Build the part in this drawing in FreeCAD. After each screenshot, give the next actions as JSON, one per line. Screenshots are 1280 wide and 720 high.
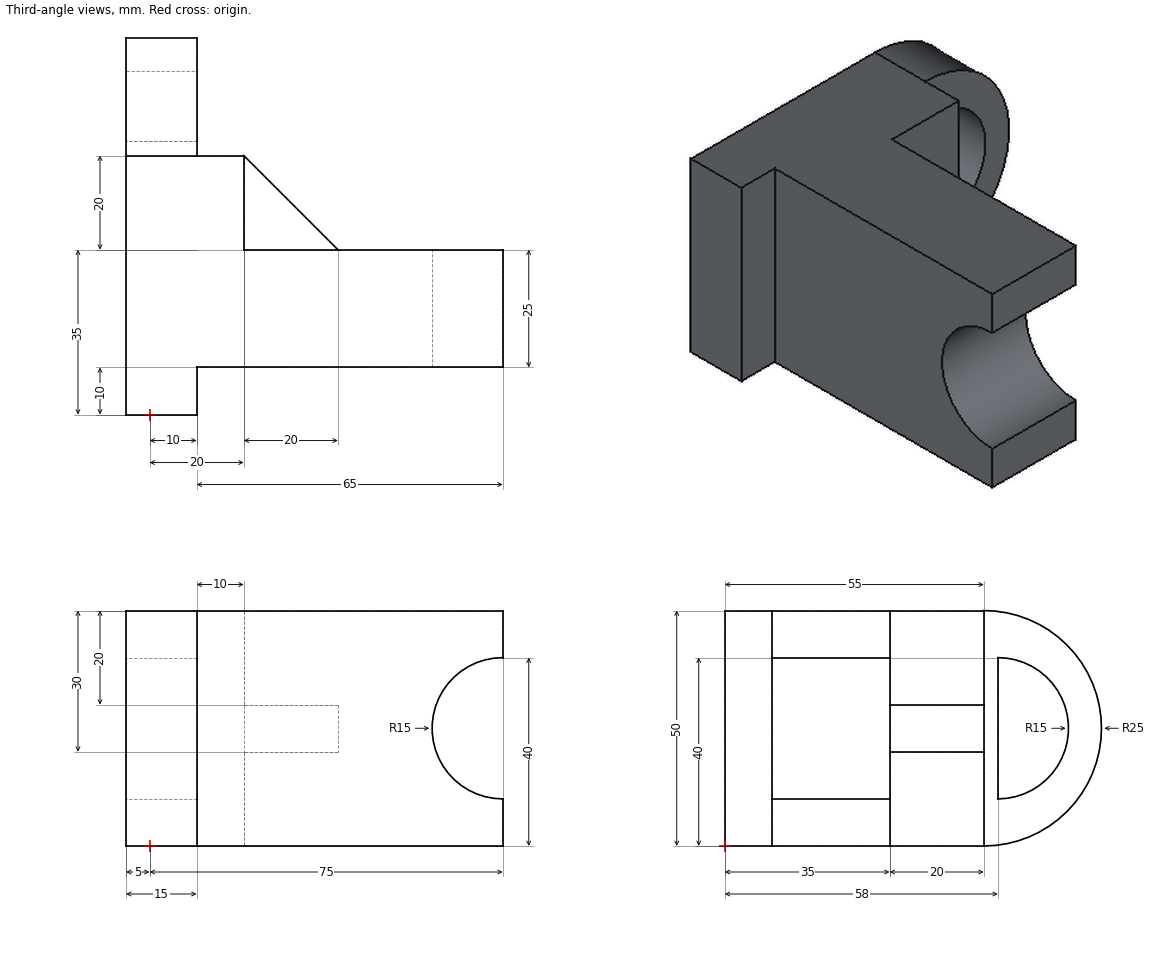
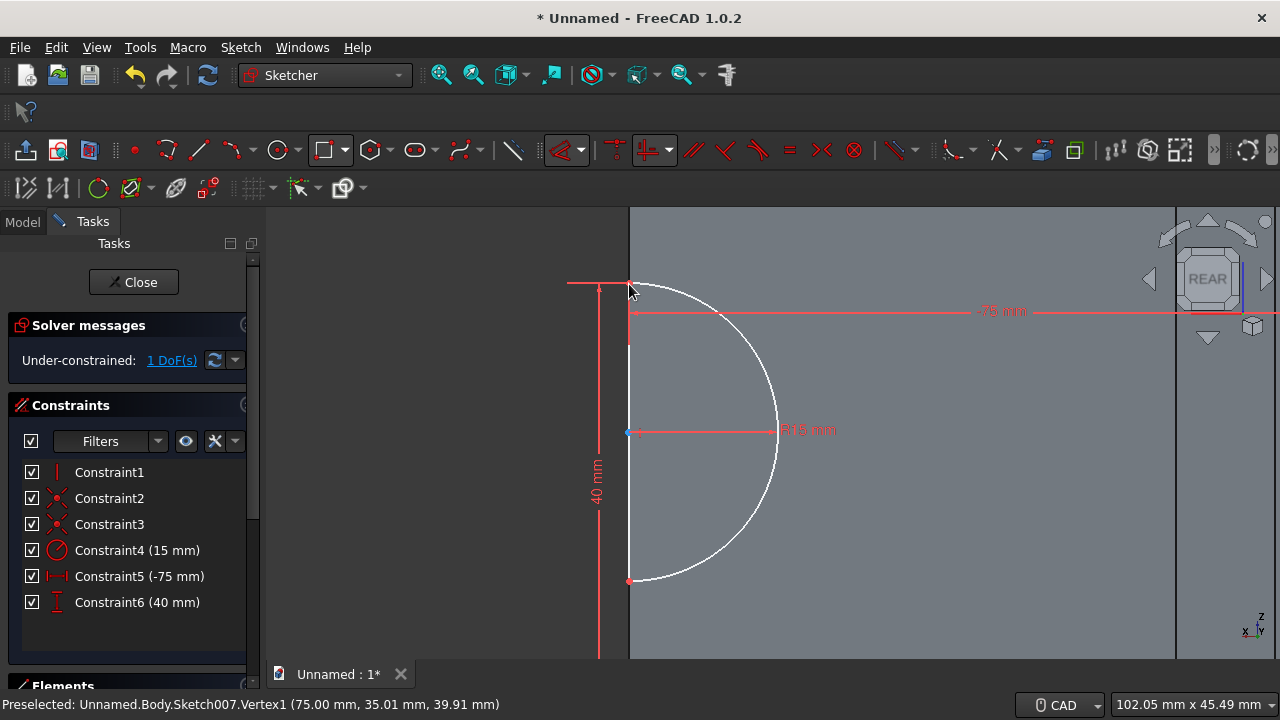
{"action": "left_click", "coordinate": [629, 432]}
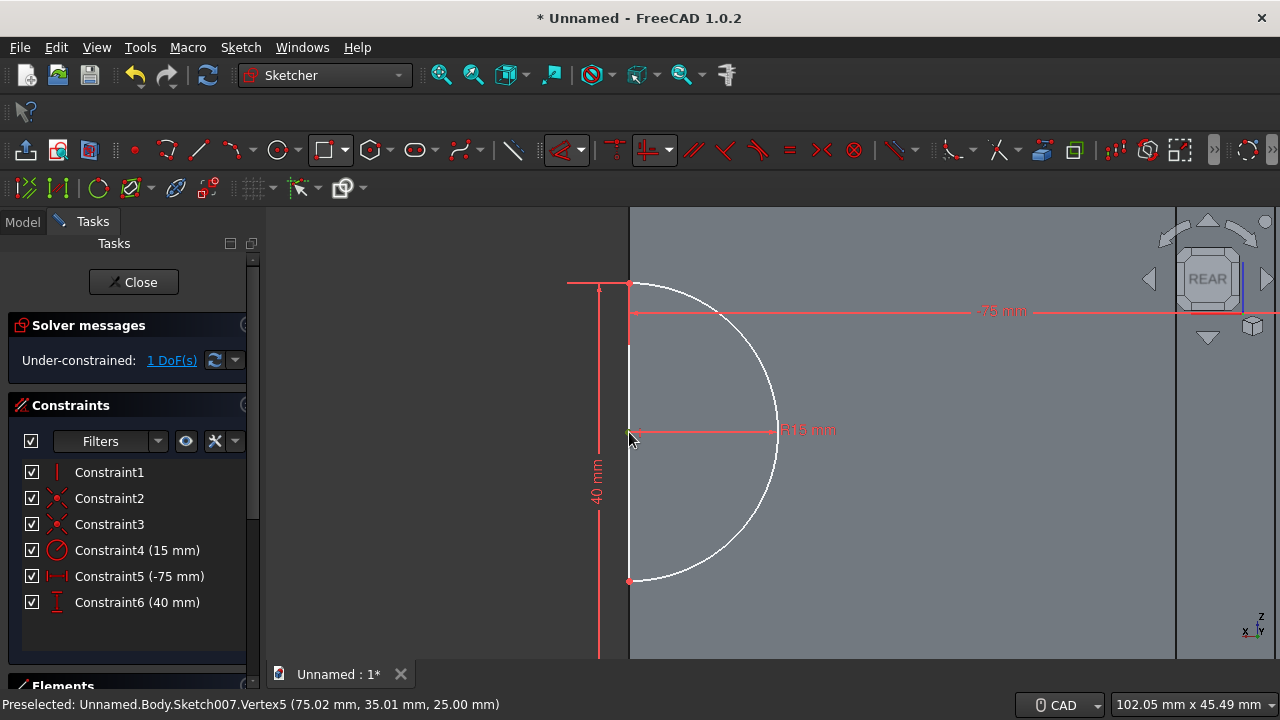
{"action": "key", "text": "l"}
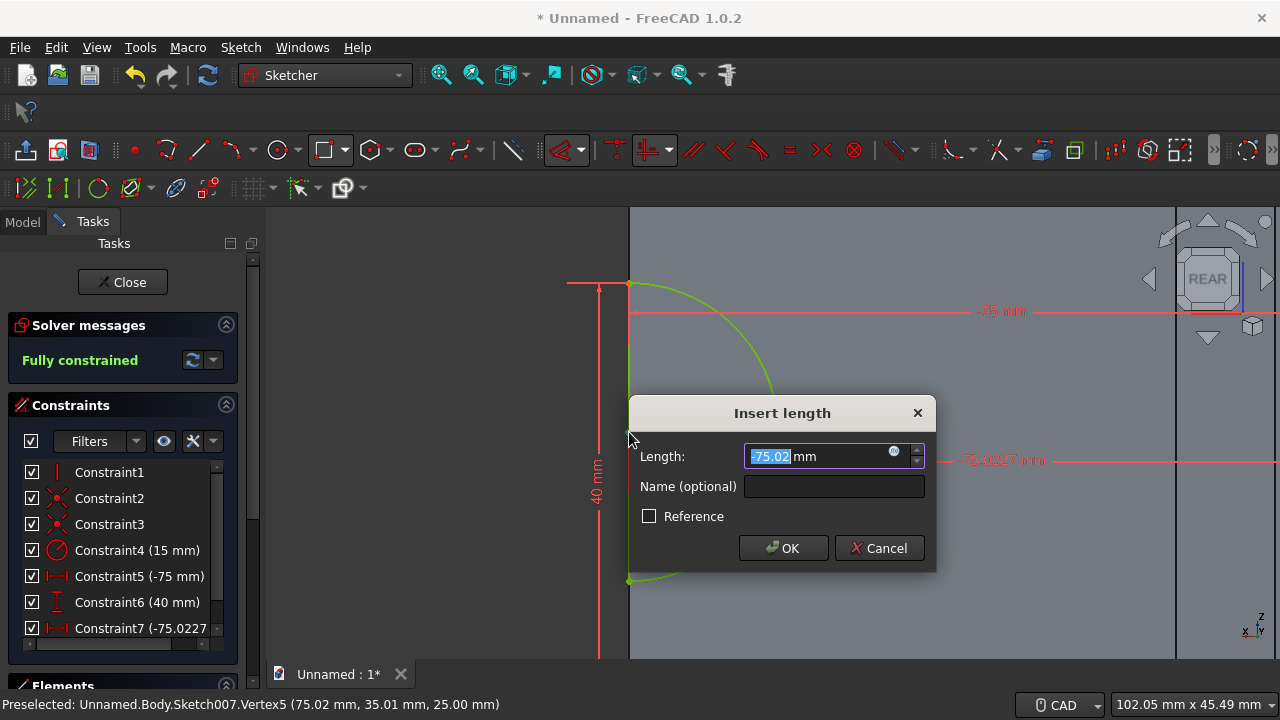
{"action": "type", "text": "-75"}
{"action": "key", "text": "Return"}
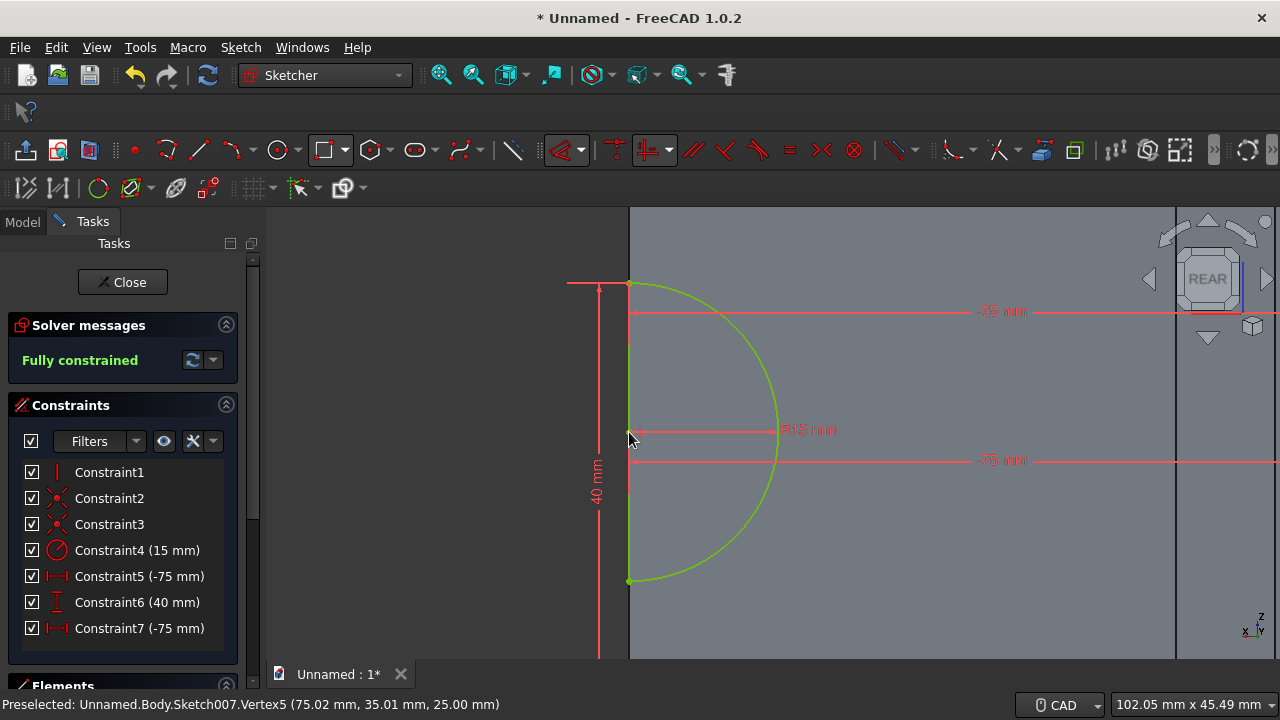
{"action": "left_click", "coordinate": [123, 282]}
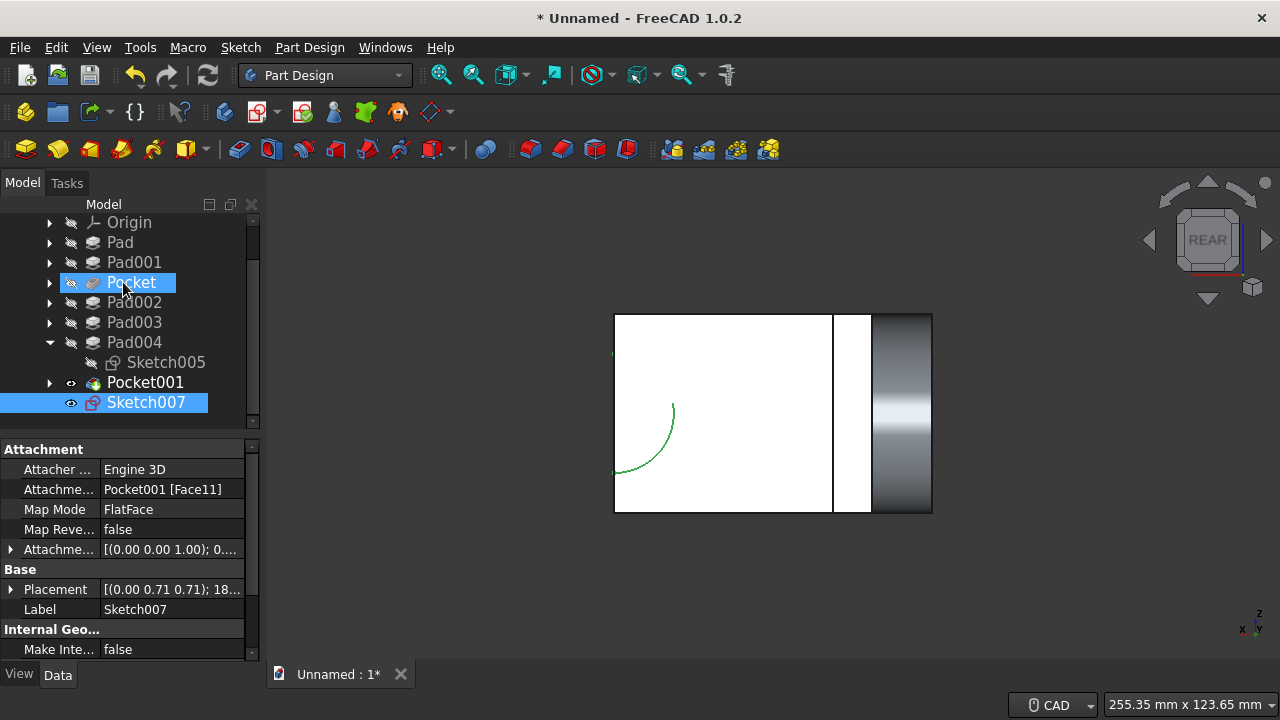
{"action": "left_click", "coordinate": [240, 150]}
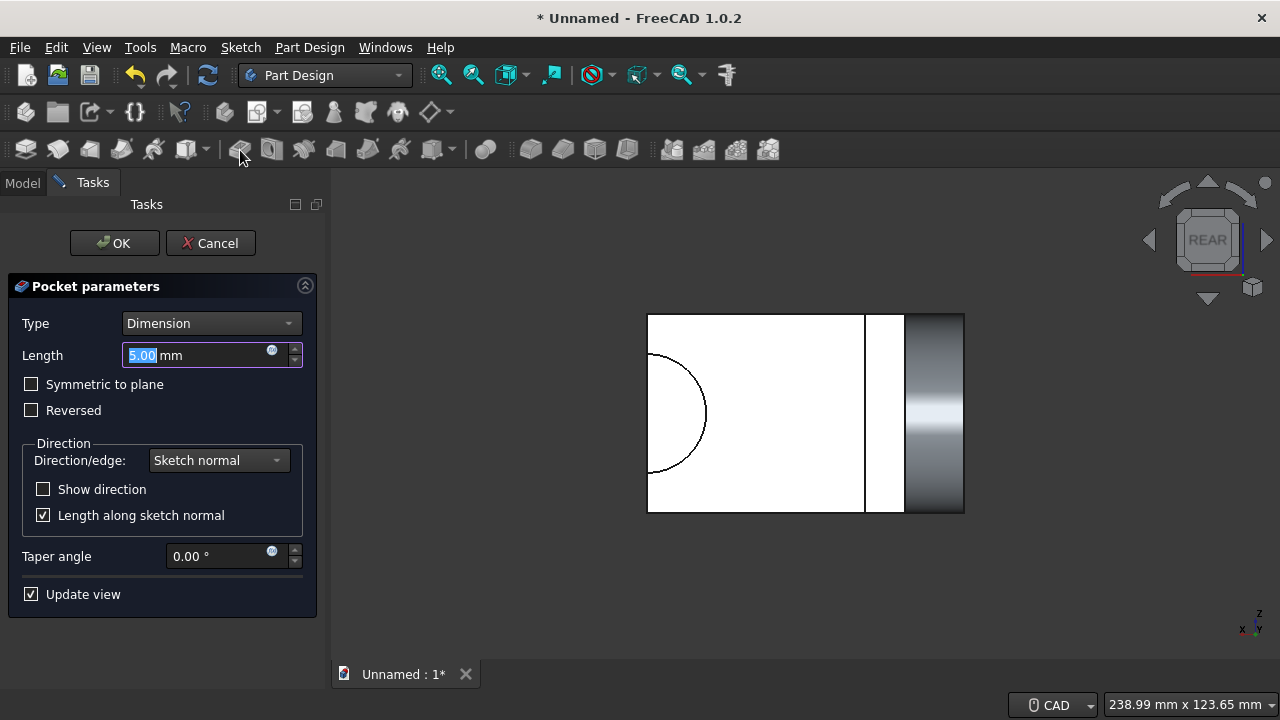
{"action": "type", "text": "25"}
{"action": "key", "text": "Tab"}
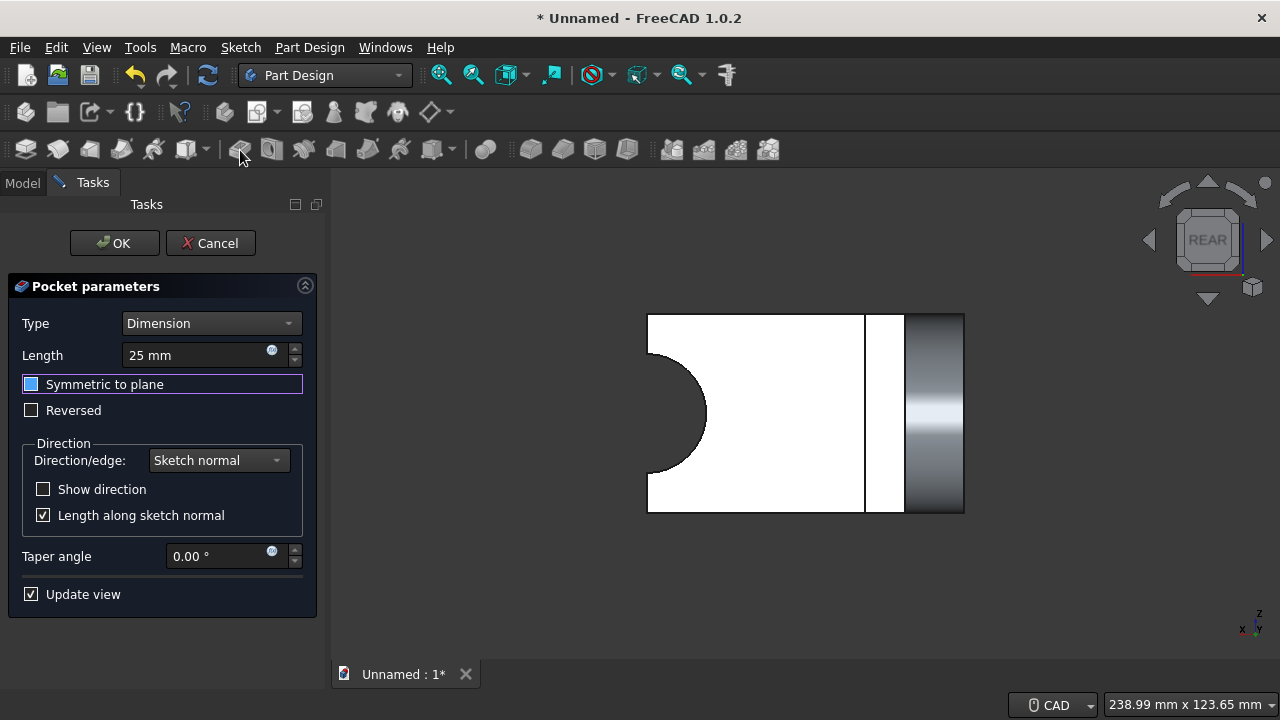
{"action": "left_click", "coordinate": [115, 243]}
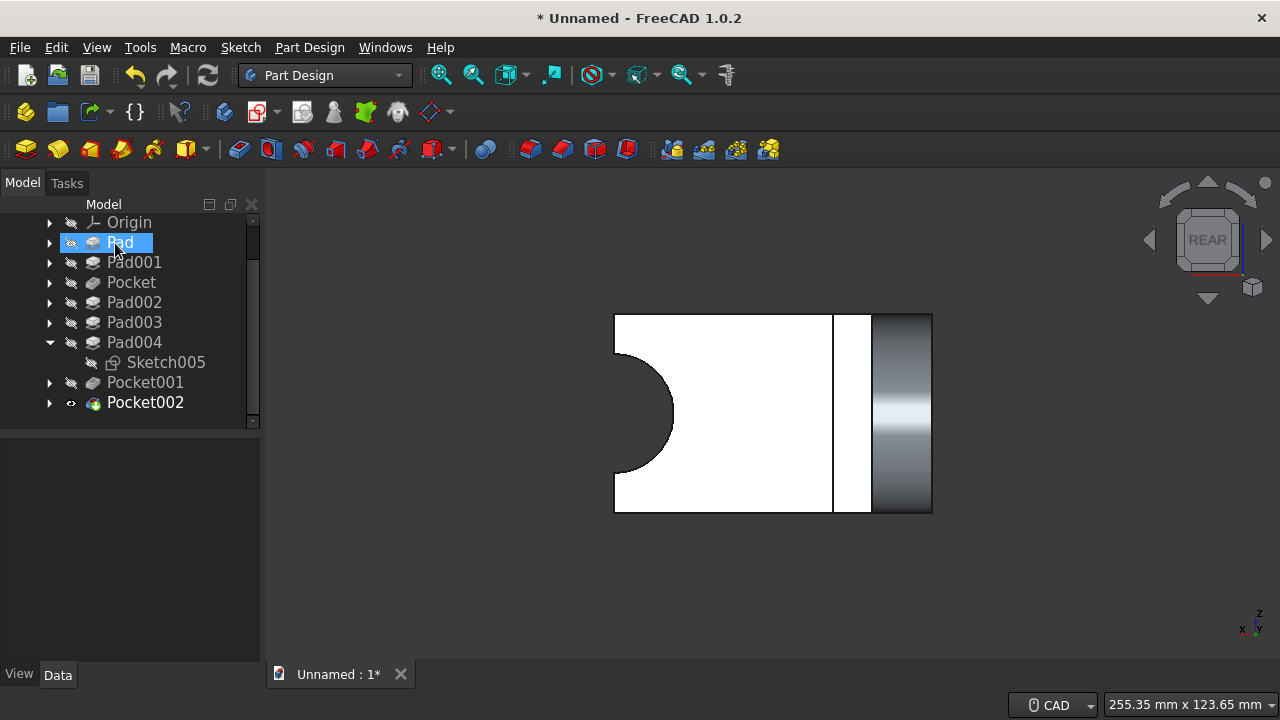
{"action": "left_click", "coordinate": [442, 76]}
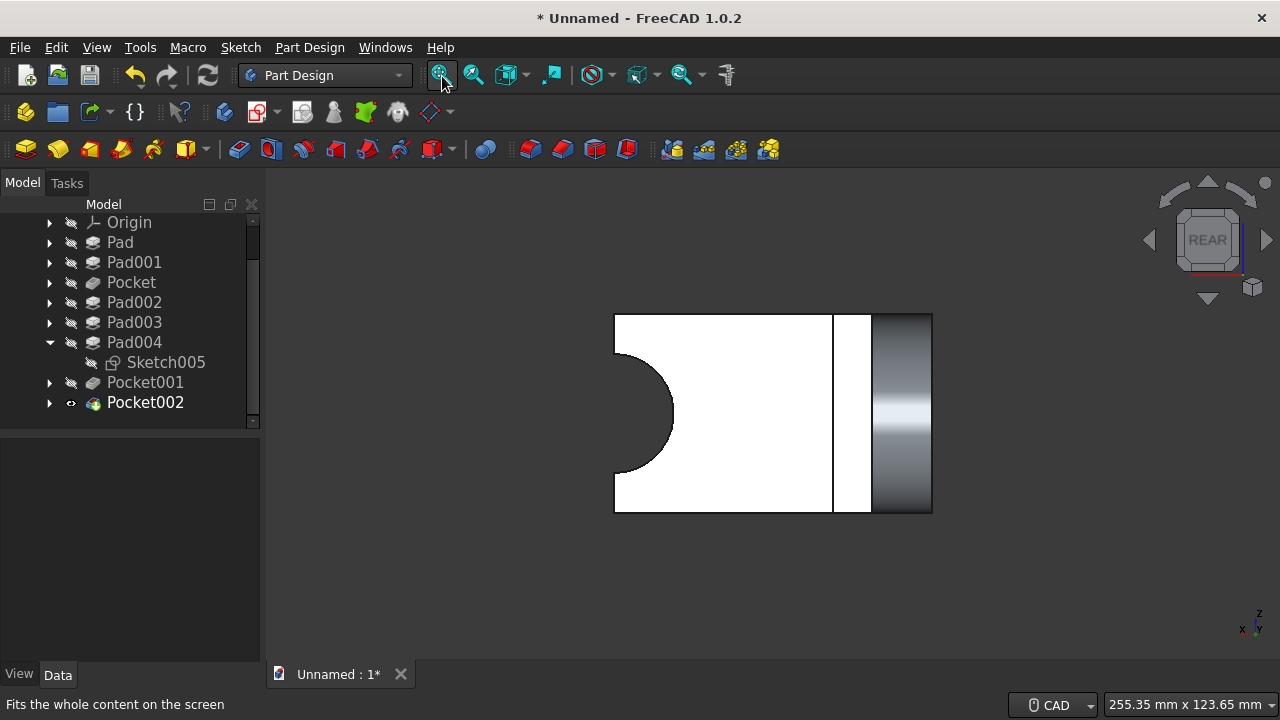
{"action": "key", "text": "0"}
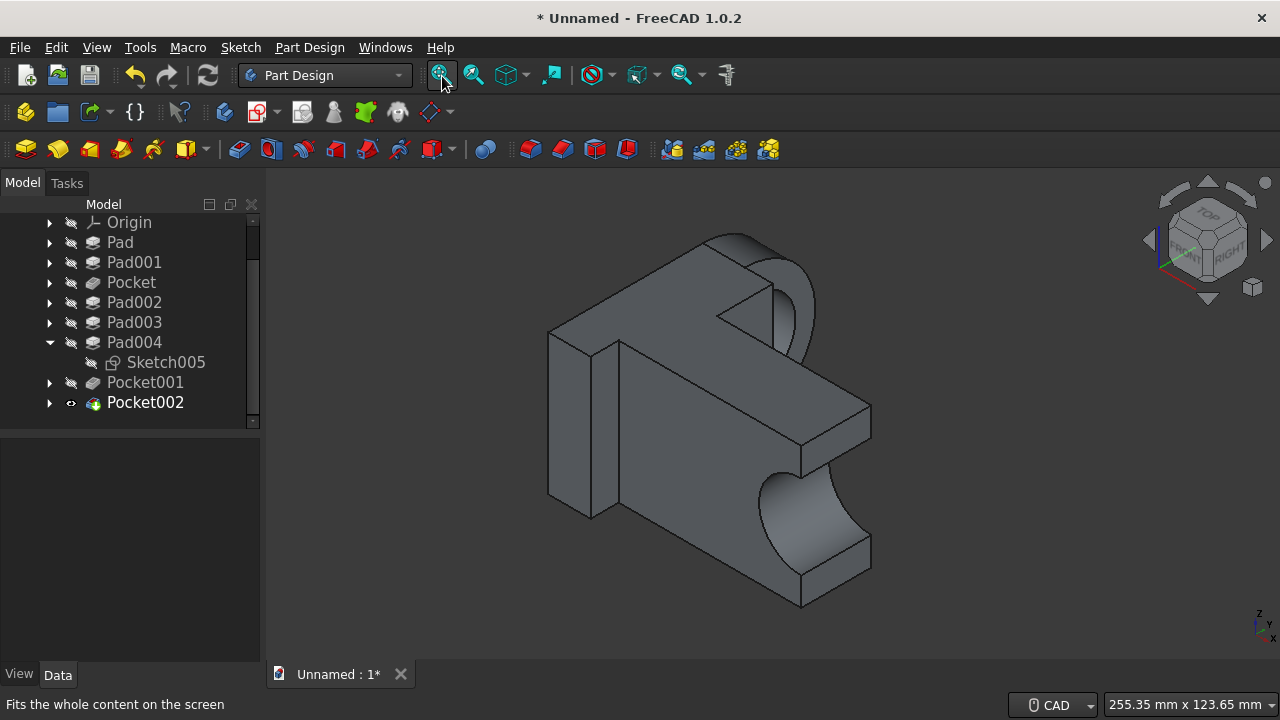
{"action": "left_click", "coordinate": [674, 315]}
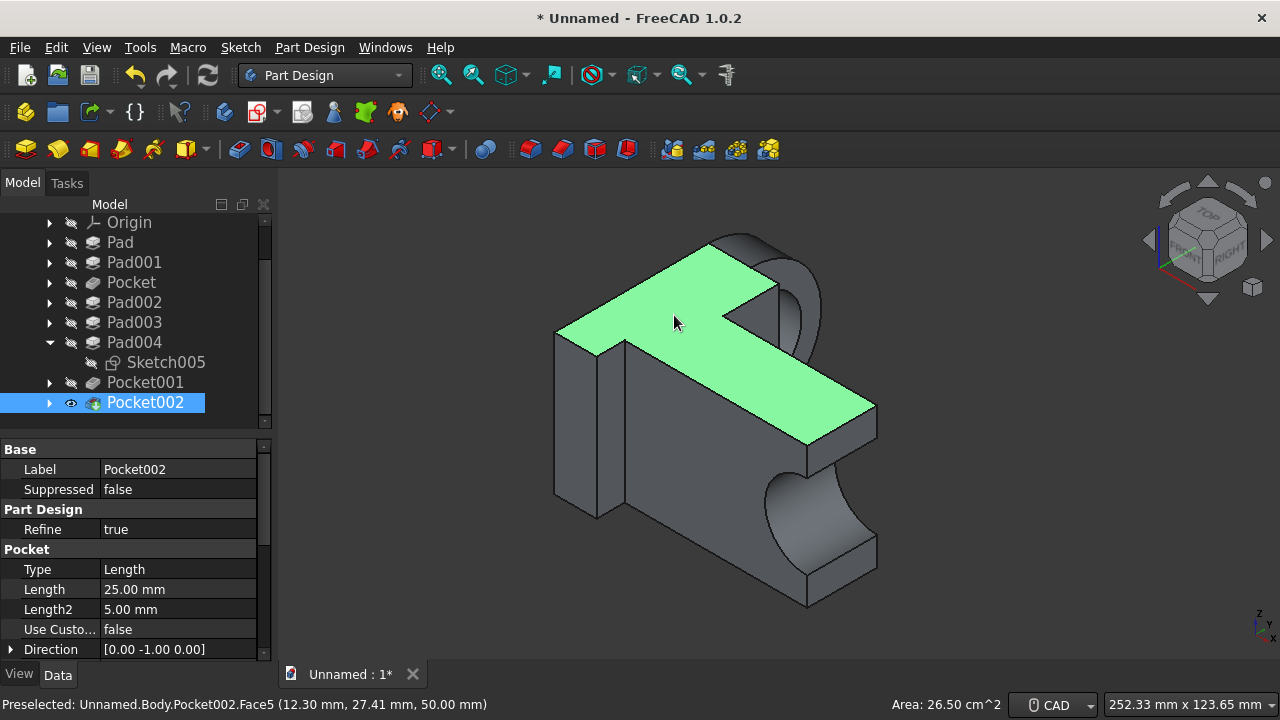
{"action": "left_click", "coordinate": [258, 112]}